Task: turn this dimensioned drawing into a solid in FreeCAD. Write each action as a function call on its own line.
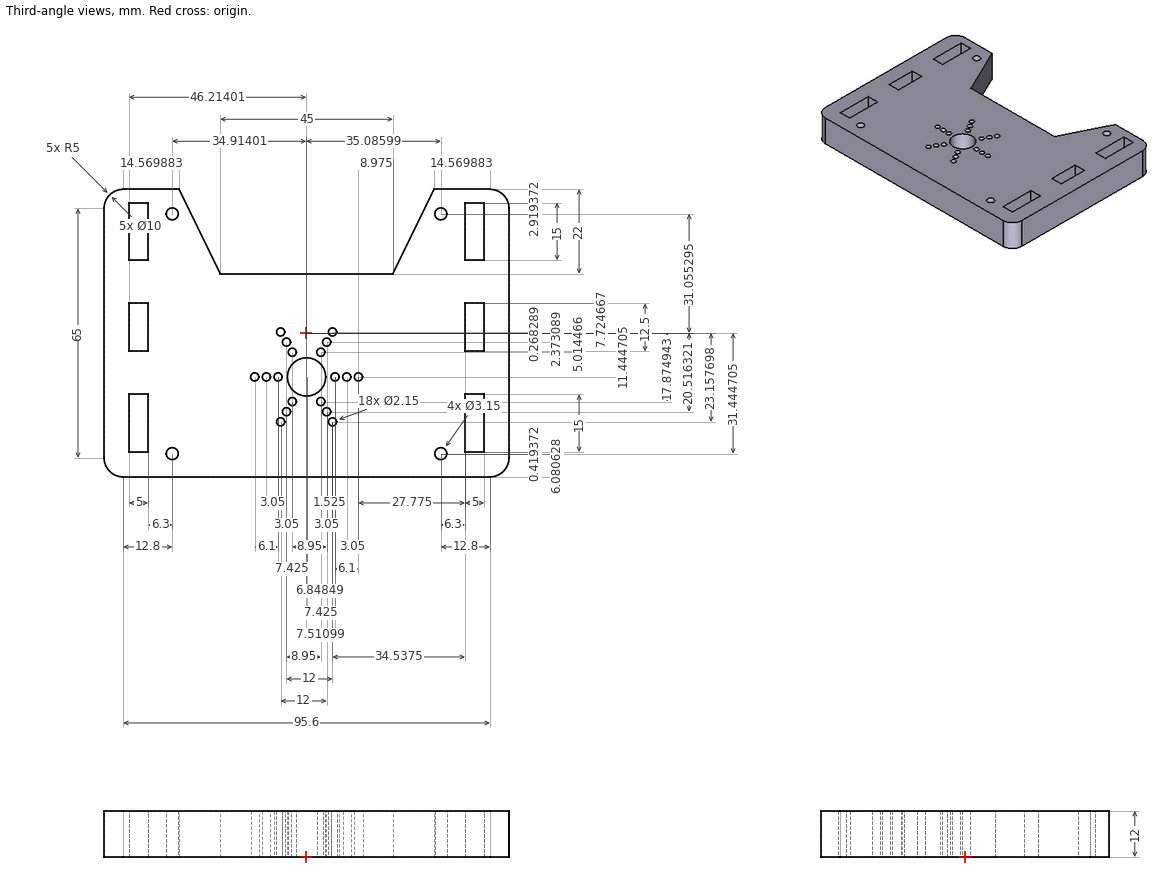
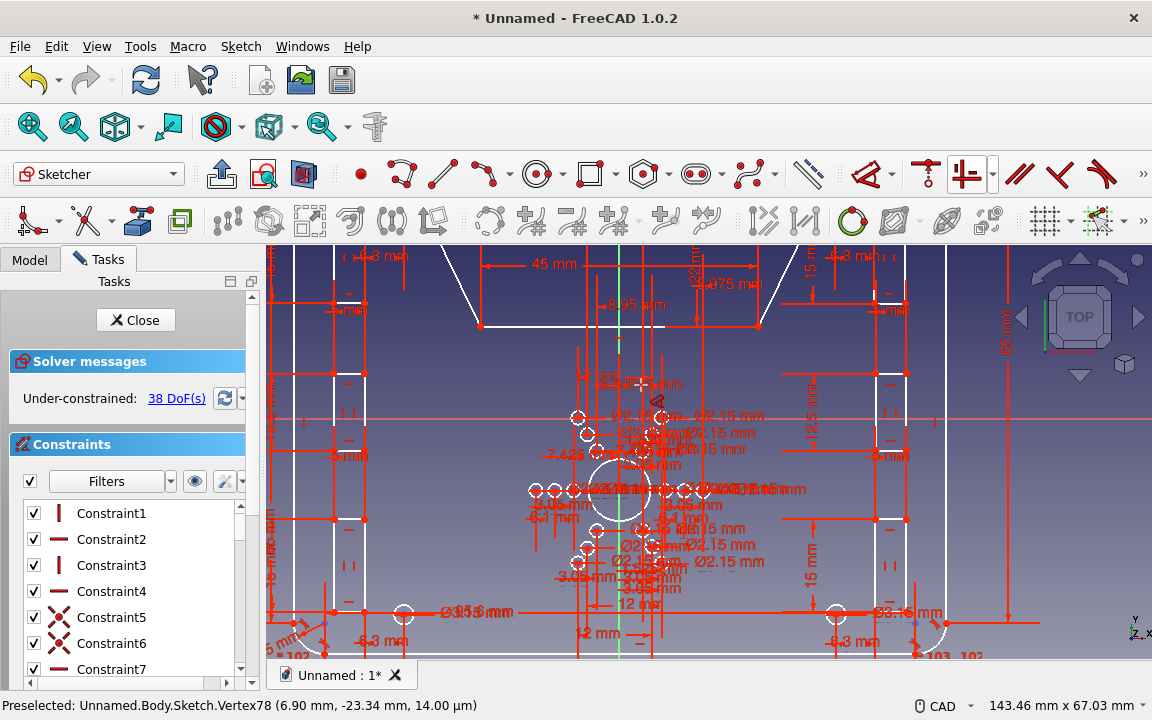
click(665, 491)
click(632, 549)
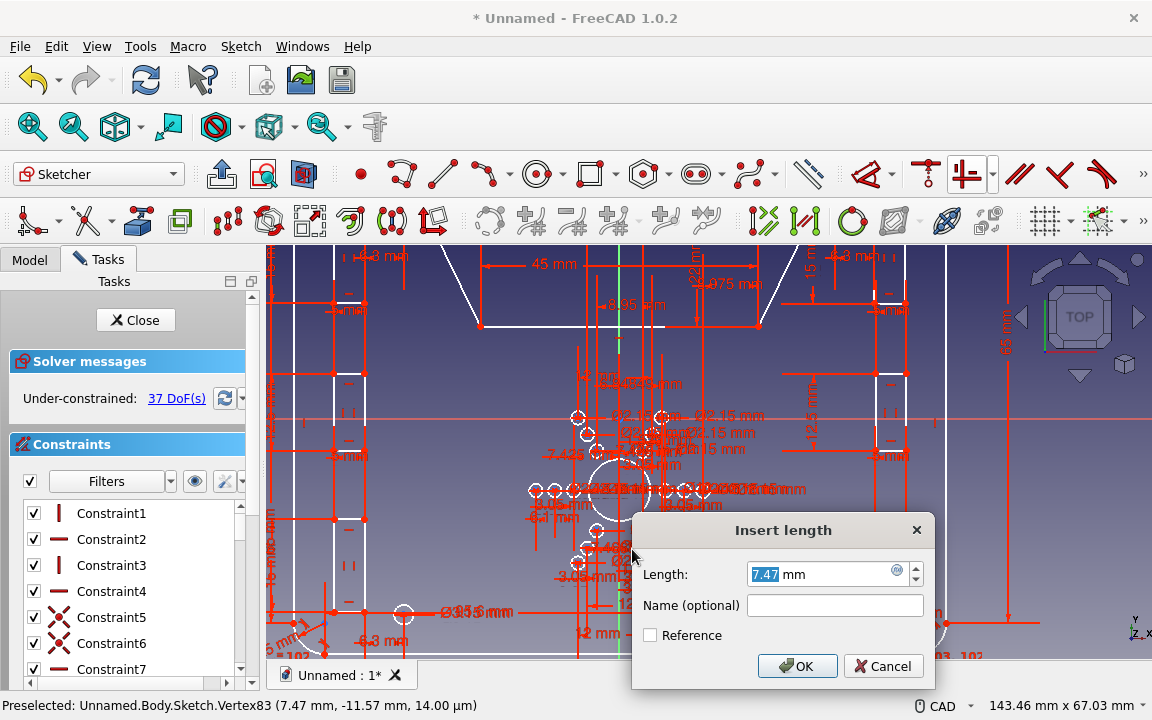
text(7.51099)
key(Return)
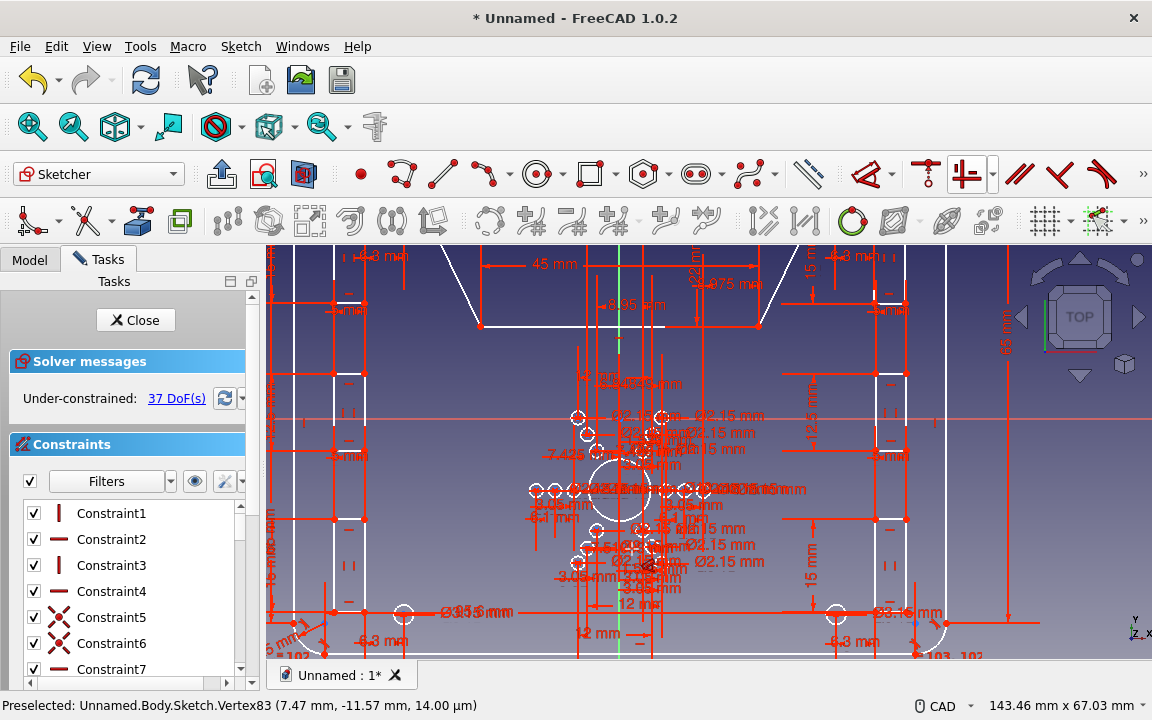
click(875, 519)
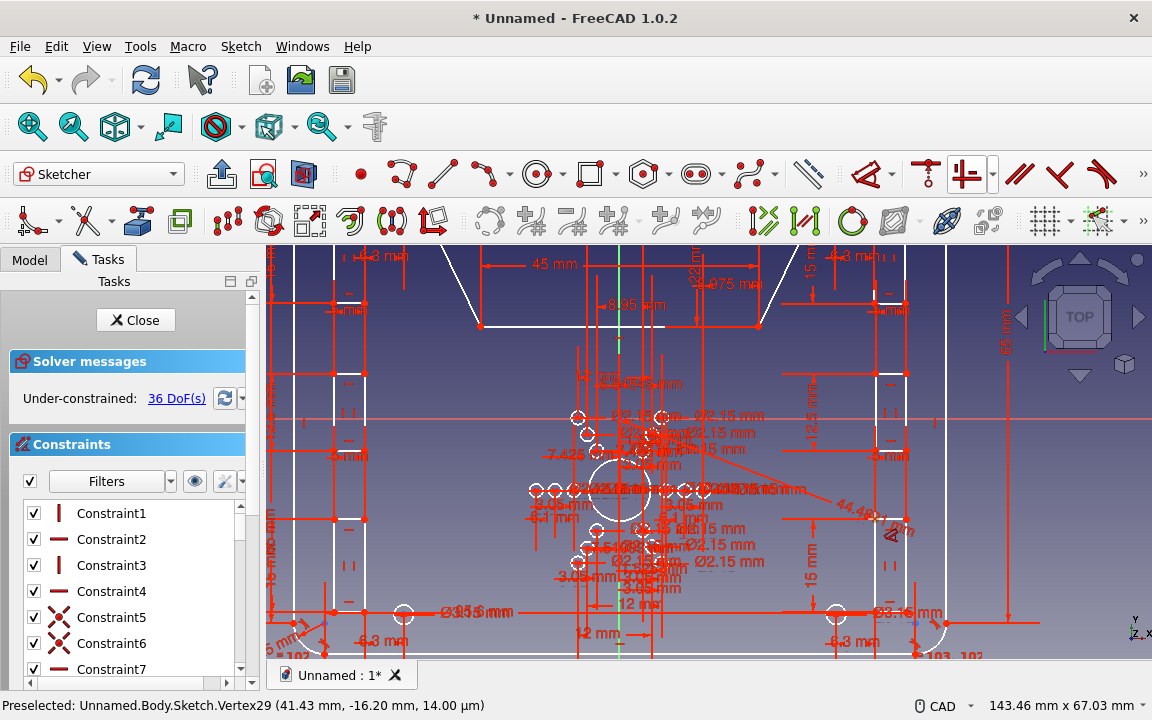
click(703, 491)
click(789, 553)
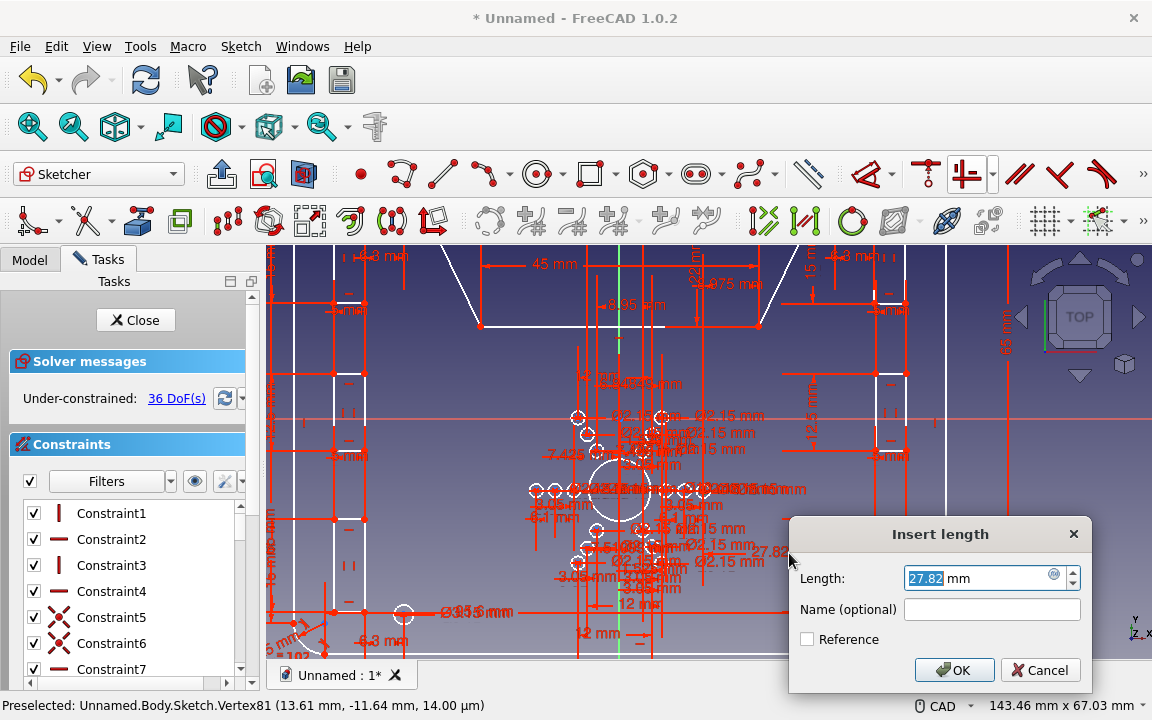
text(27.775)
key(Return)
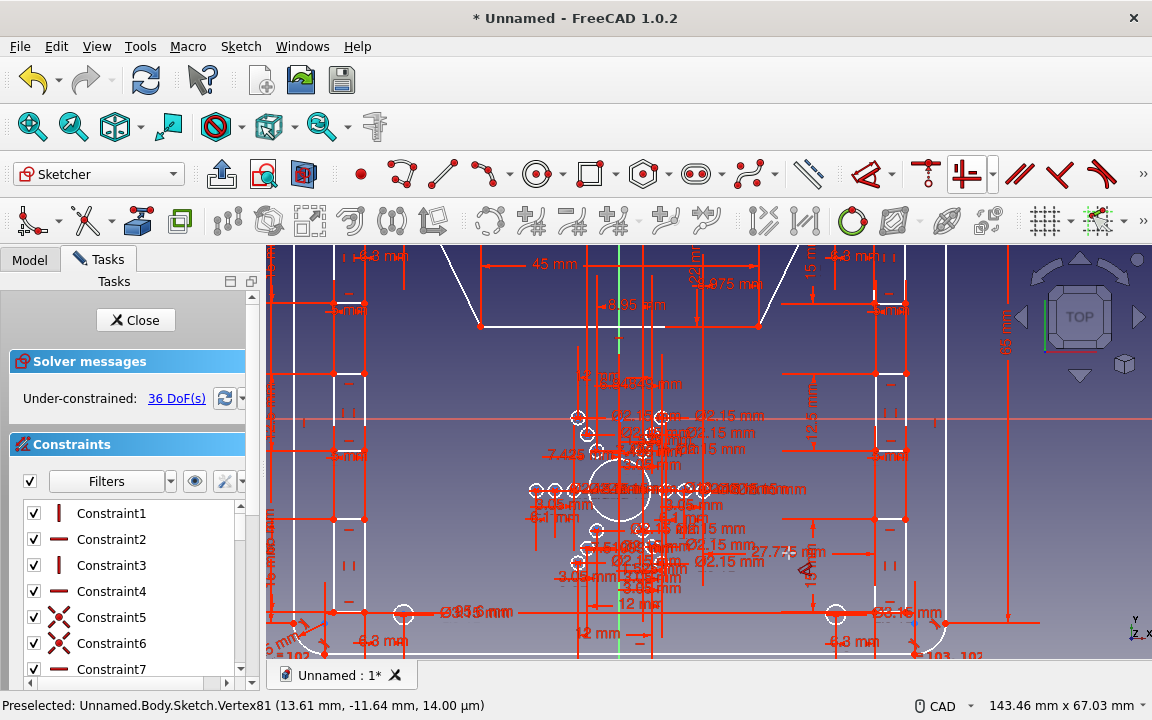
scroll(643, 451, up, 2)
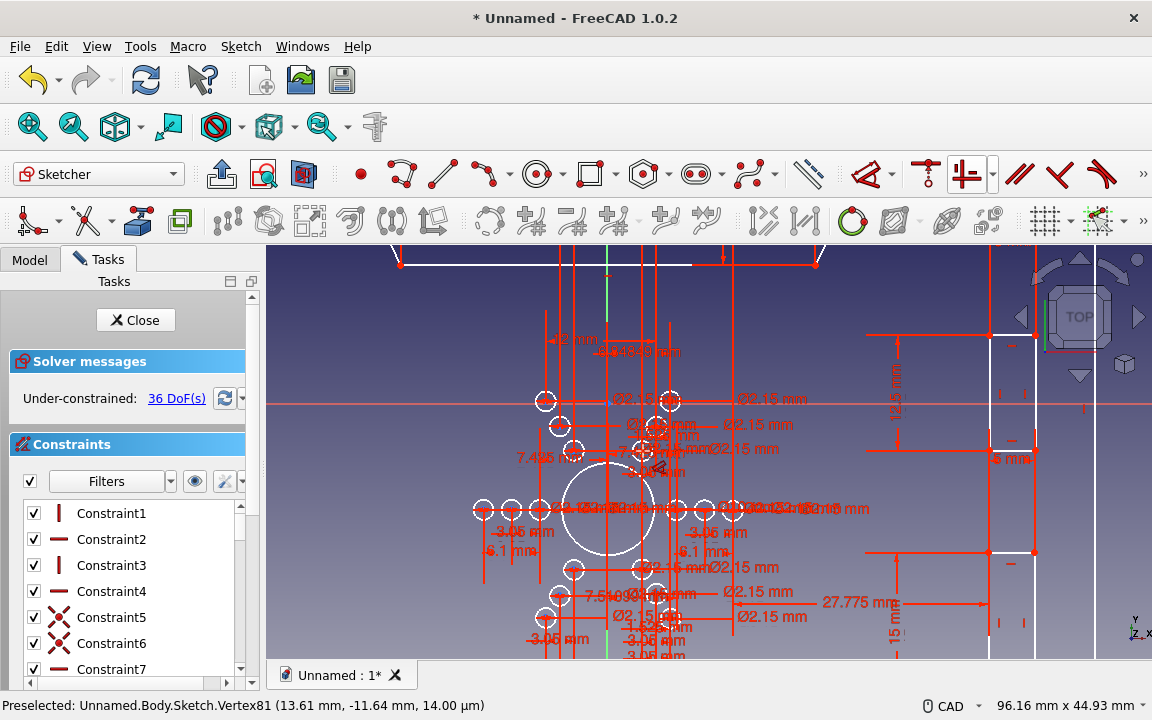
click(642, 451)
click(525, 427)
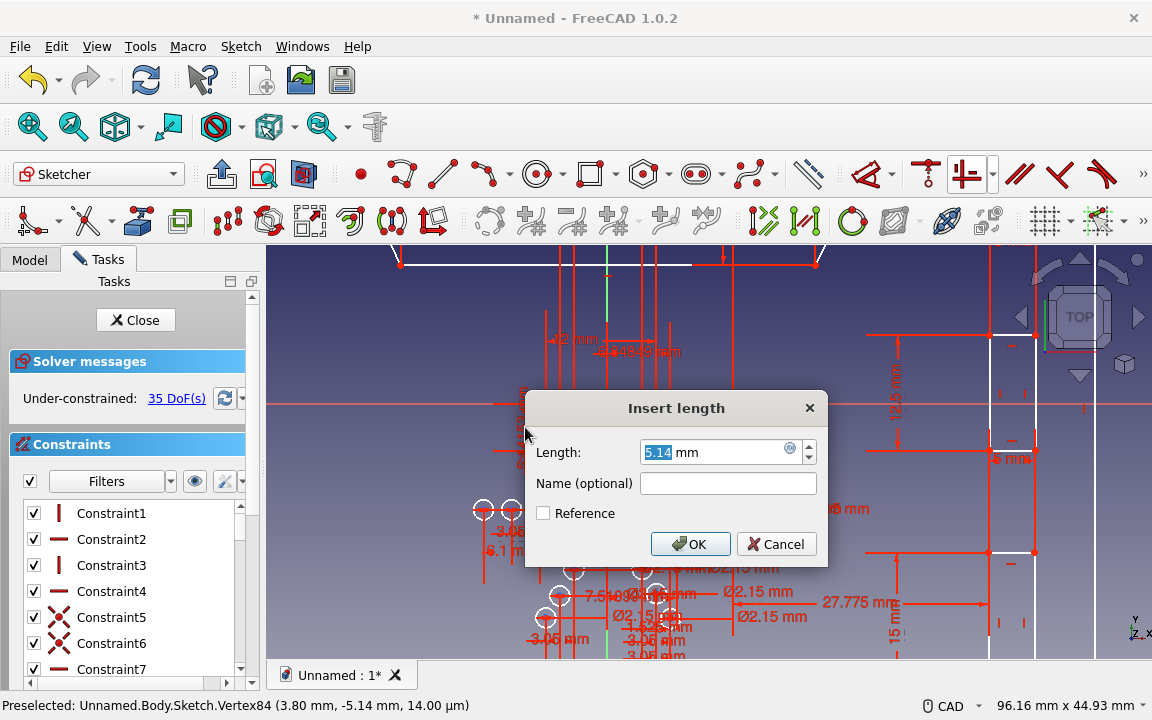
text(5.014466)
key(Return)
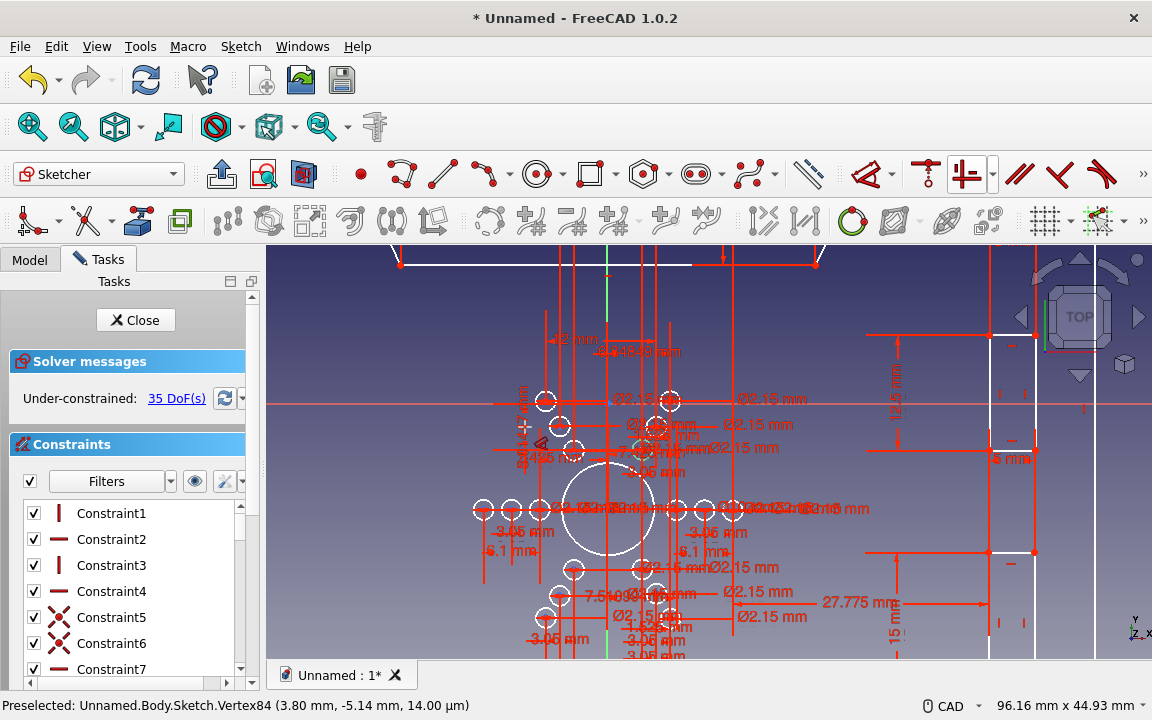
scroll(670, 401, up, 14)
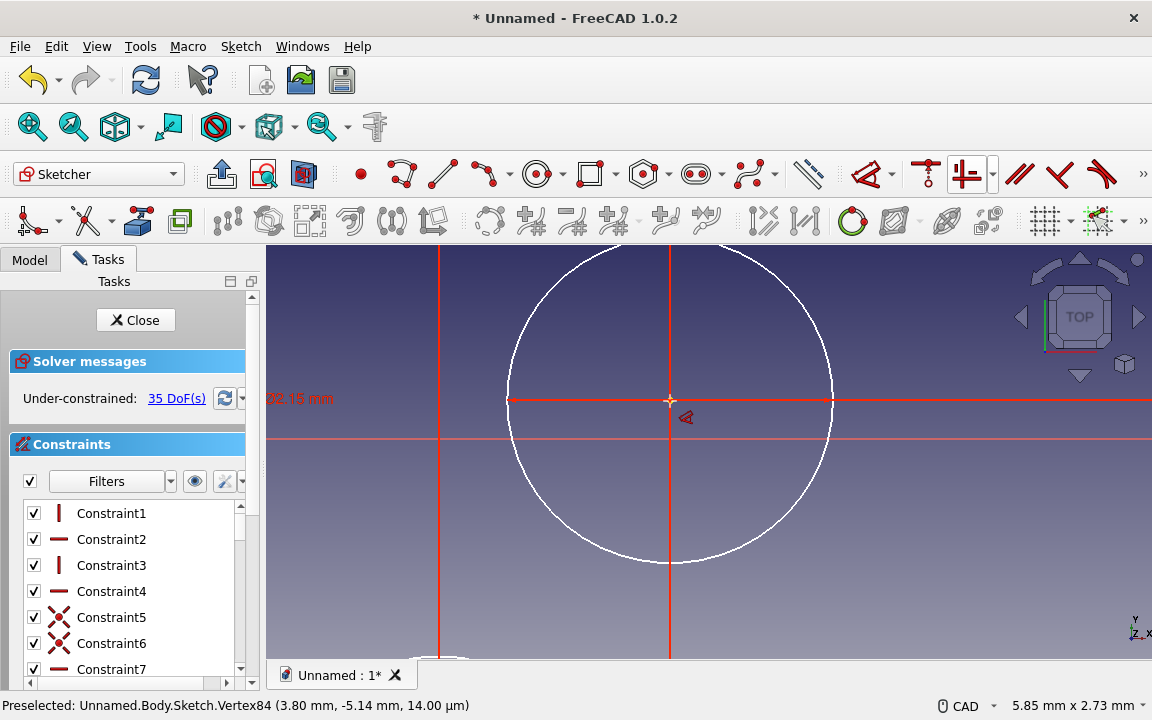
click(670, 400)
click(704, 420)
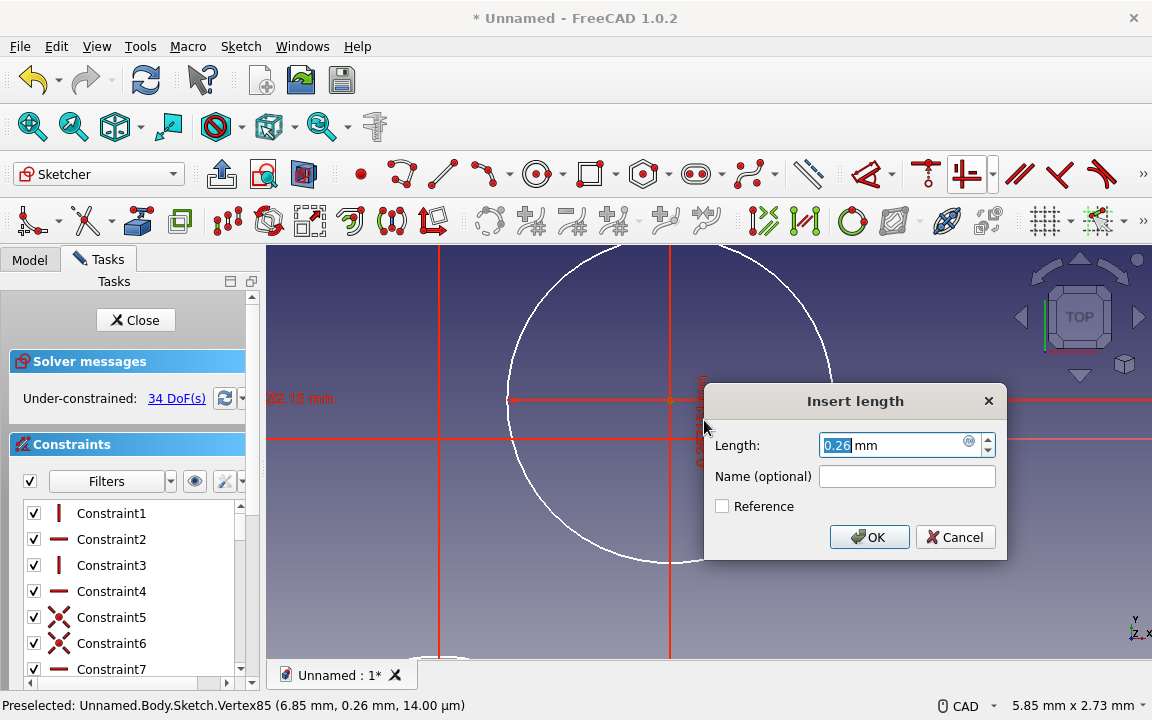
text(0.268289)
key(Return)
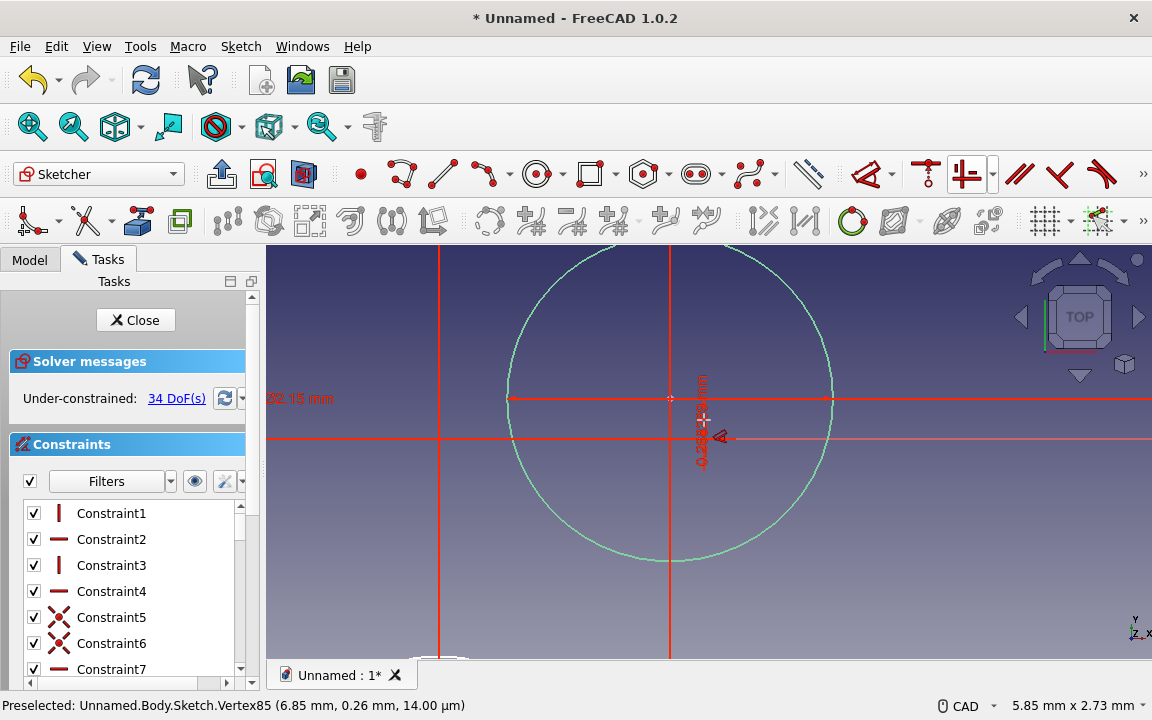
scroll(640, 452, down, 15)